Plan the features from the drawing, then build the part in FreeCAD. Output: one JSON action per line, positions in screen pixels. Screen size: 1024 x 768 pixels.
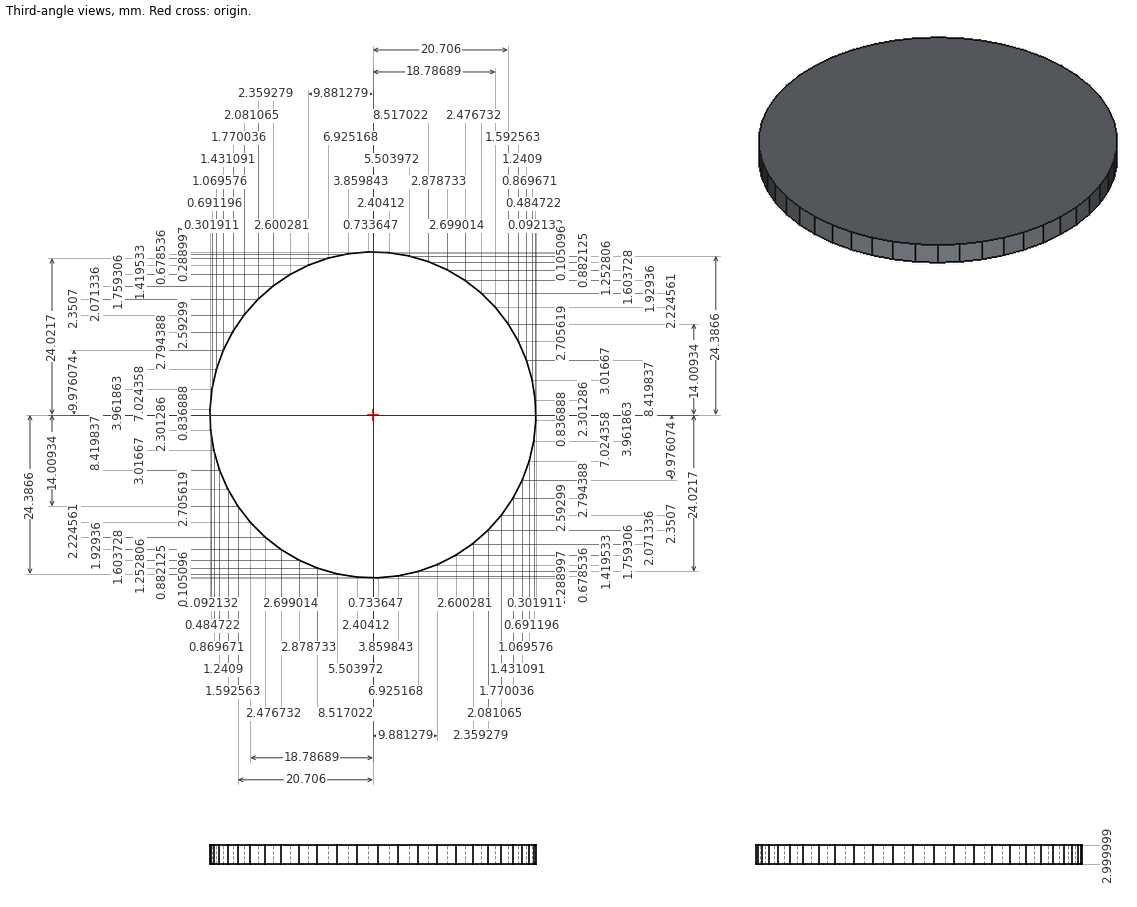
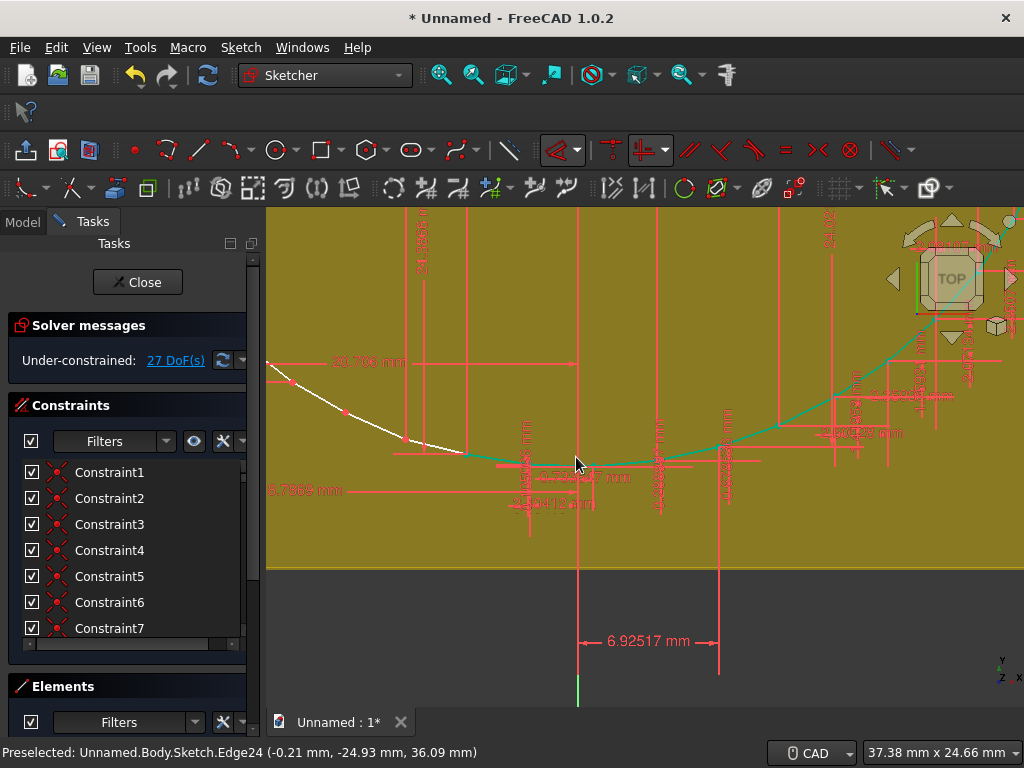
{"action": "scroll", "coordinate": [576, 671], "scroll_direction": "down", "scroll_amount": 6}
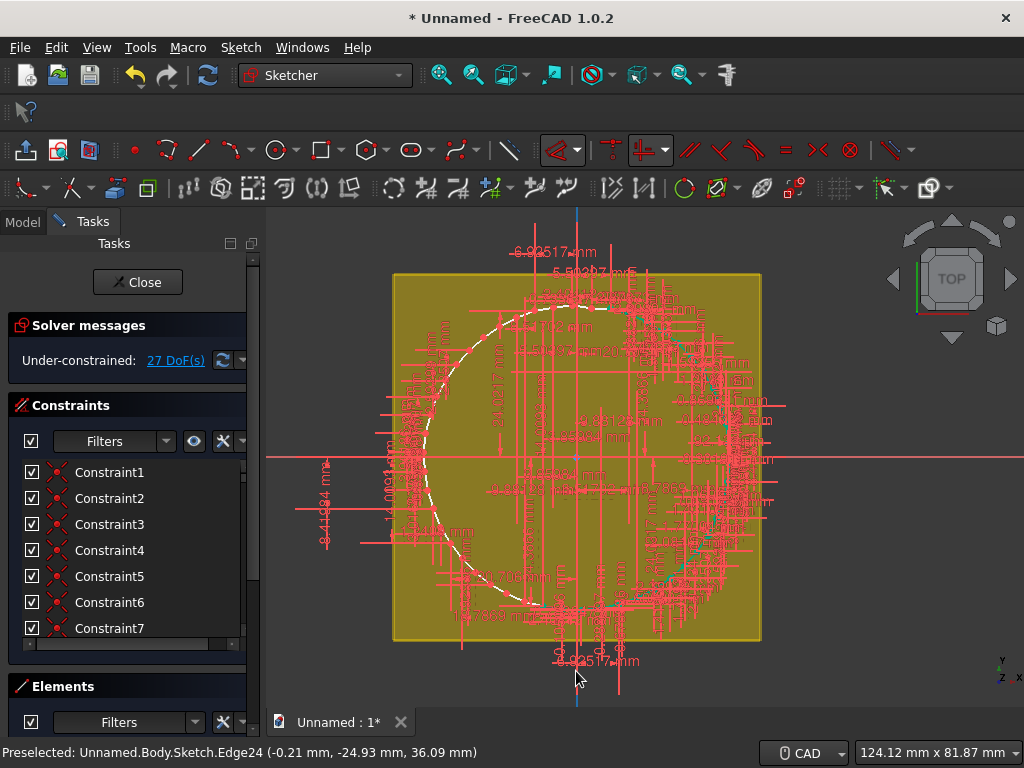
{"action": "scroll", "coordinate": [538, 605], "scroll_direction": "up", "scroll_amount": 10}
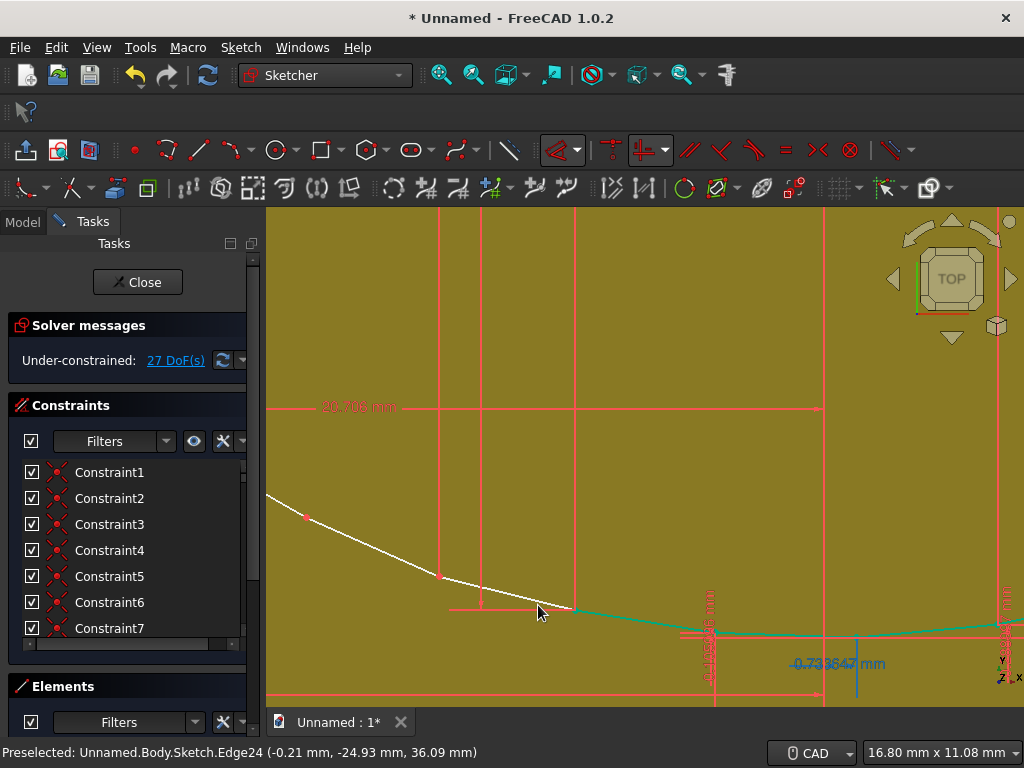
{"action": "left_click", "coordinate": [534, 600]}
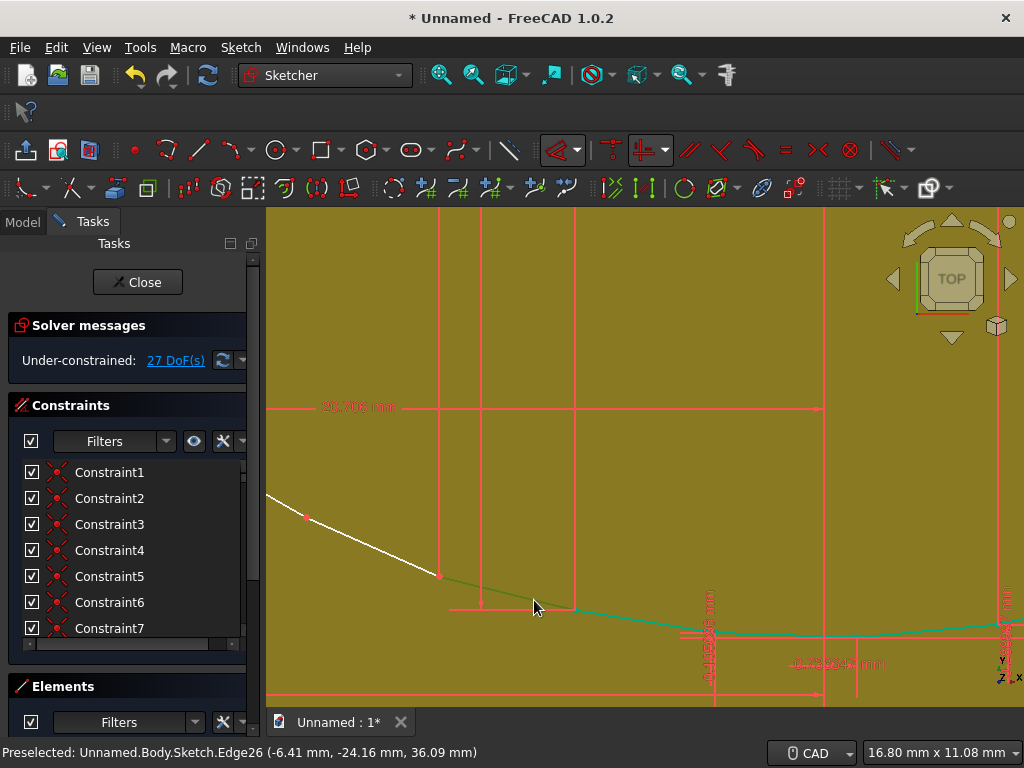
{"action": "left_click", "coordinate": [580, 150]}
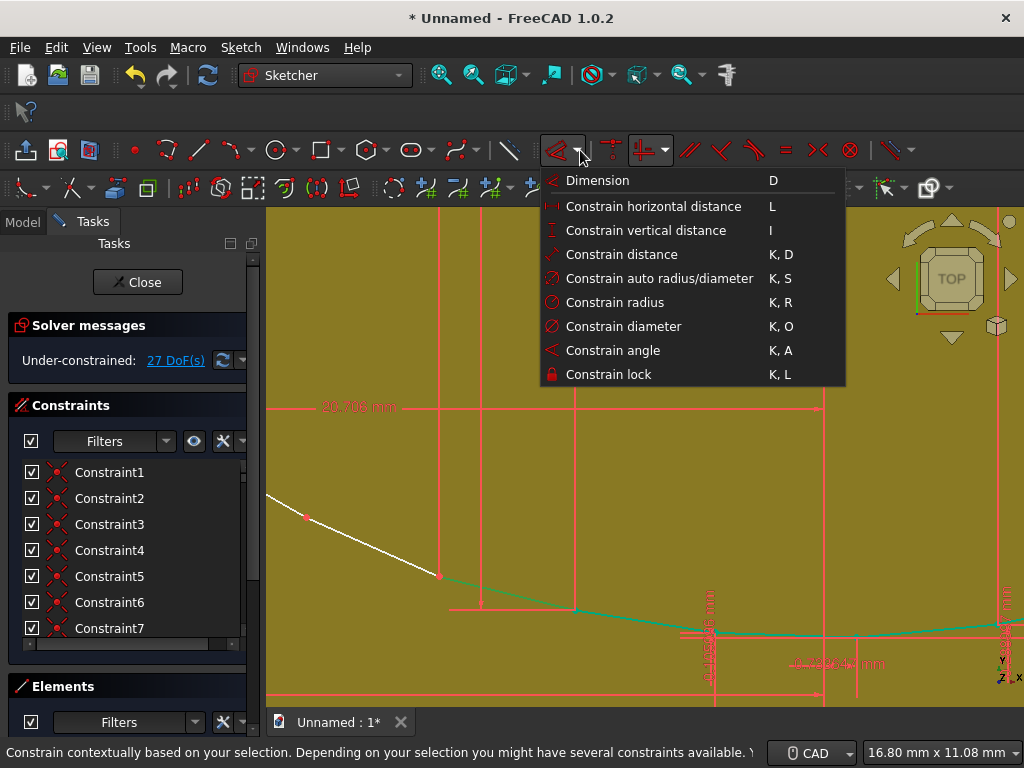
{"action": "left_click", "coordinate": [693, 230]}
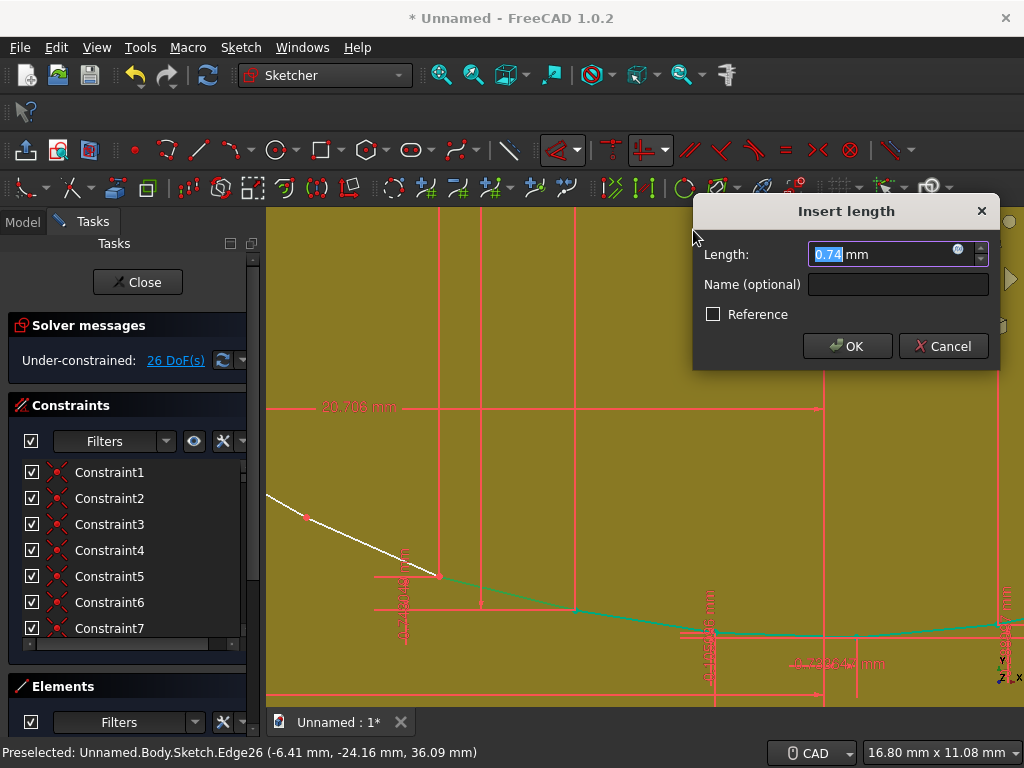
{"action": "type", "text": "0.882125"}
{"action": "key", "text": "Return"}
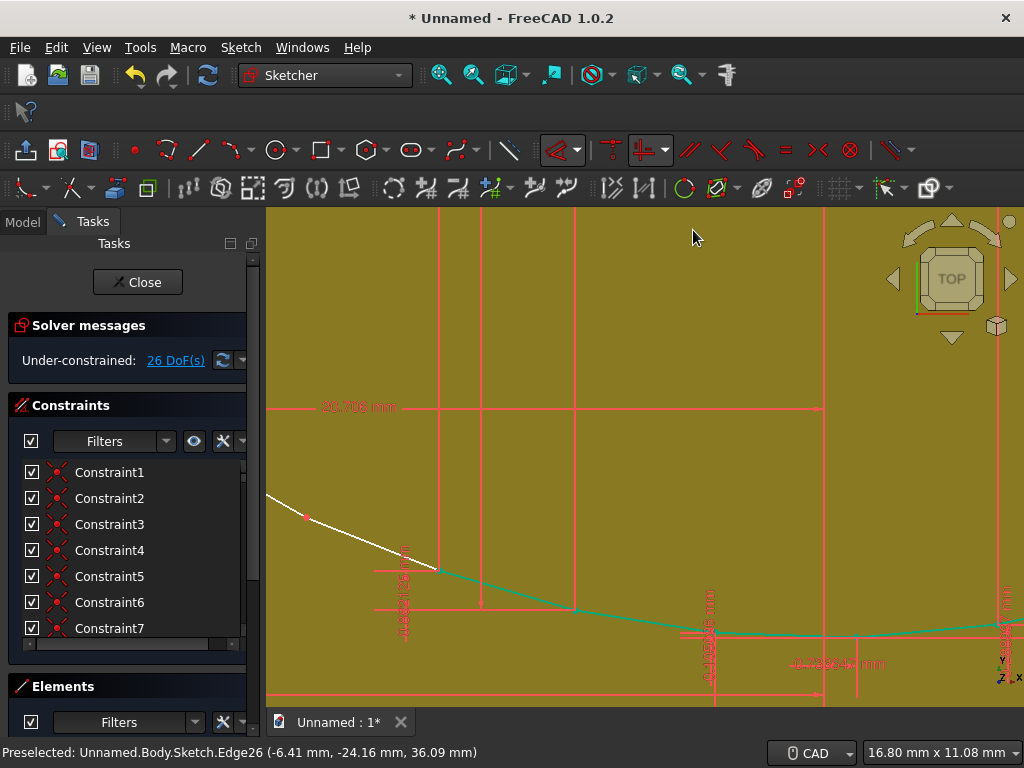
{"action": "scroll", "coordinate": [538, 605], "scroll_direction": "down", "scroll_amount": 10}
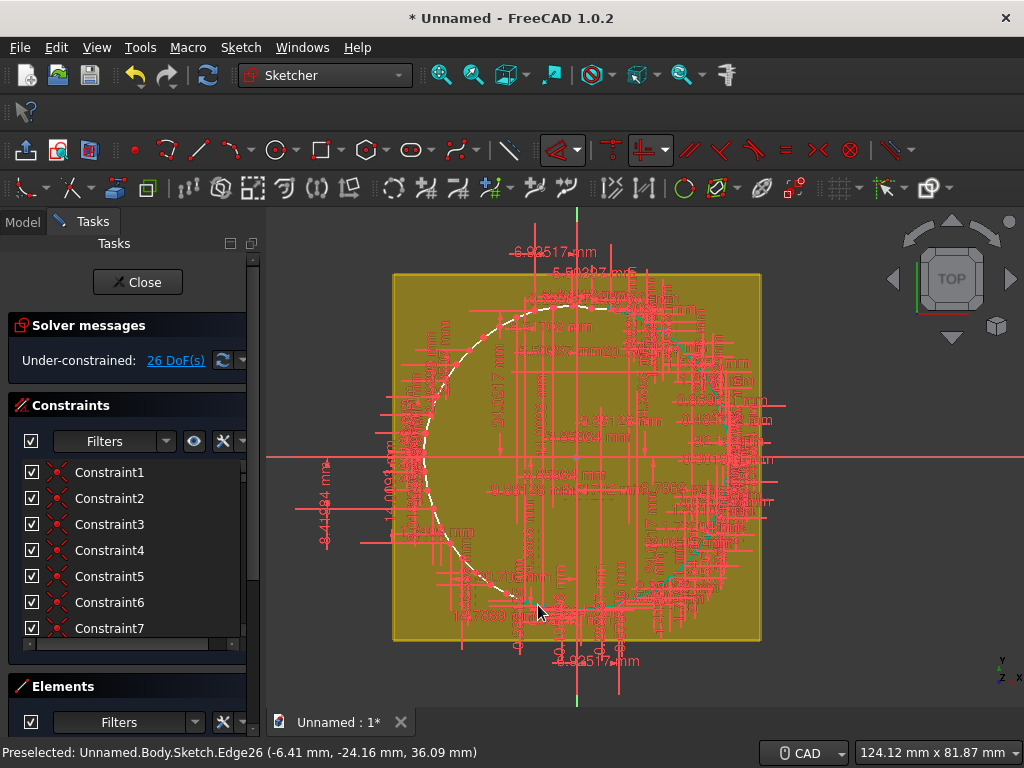
{"action": "scroll", "coordinate": [520, 599], "scroll_direction": "up", "scroll_amount": 5}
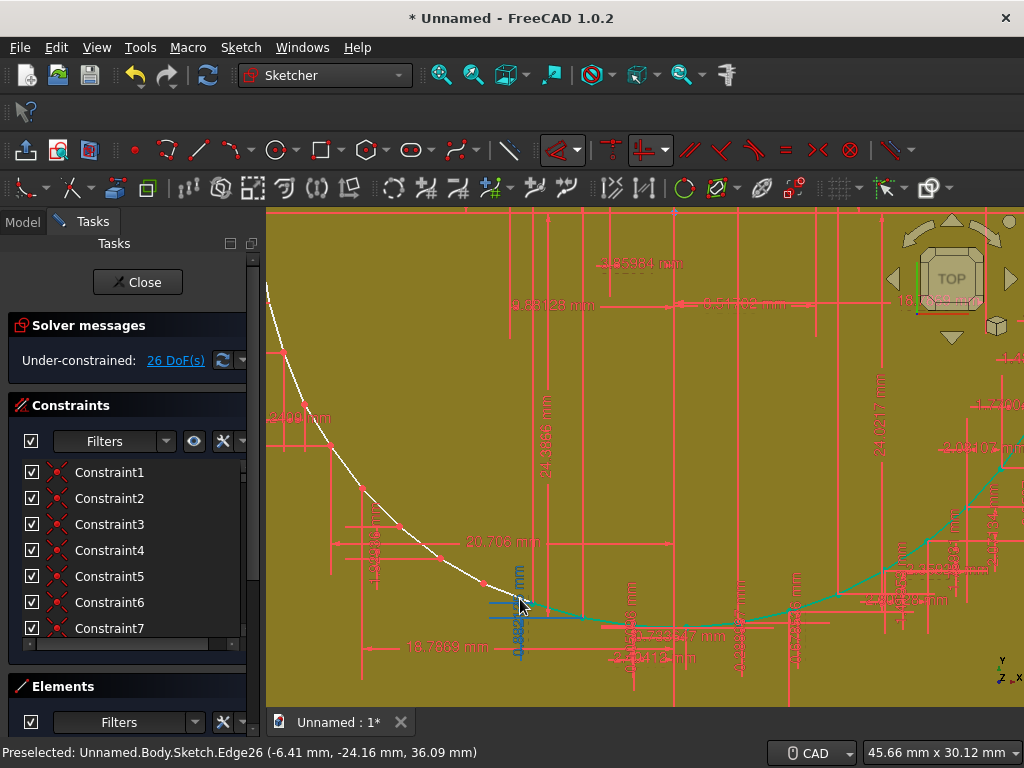
{"action": "left_click", "coordinate": [499, 590]}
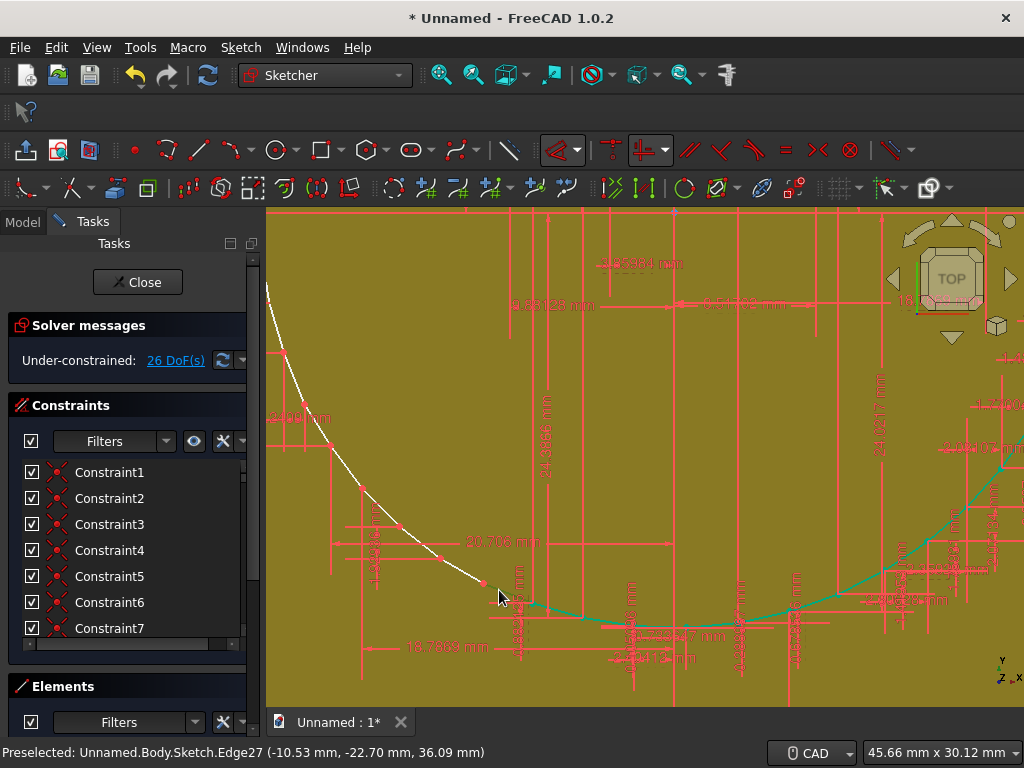
{"action": "left_click", "coordinate": [580, 150]}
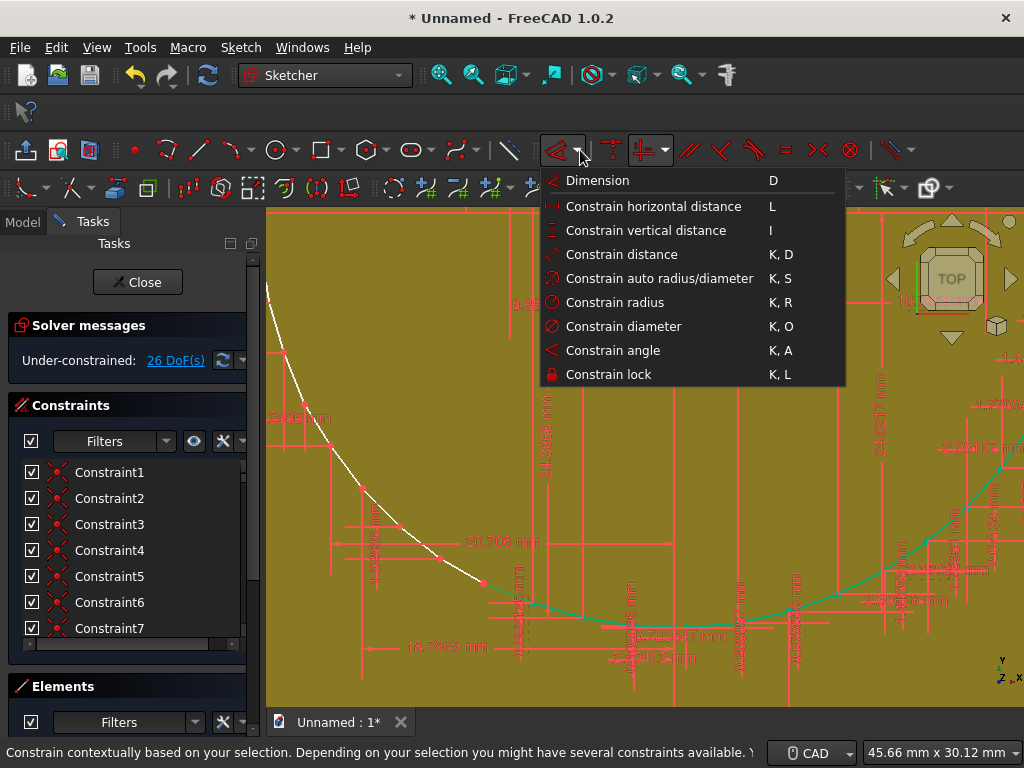
{"action": "left_click", "coordinate": [693, 206]}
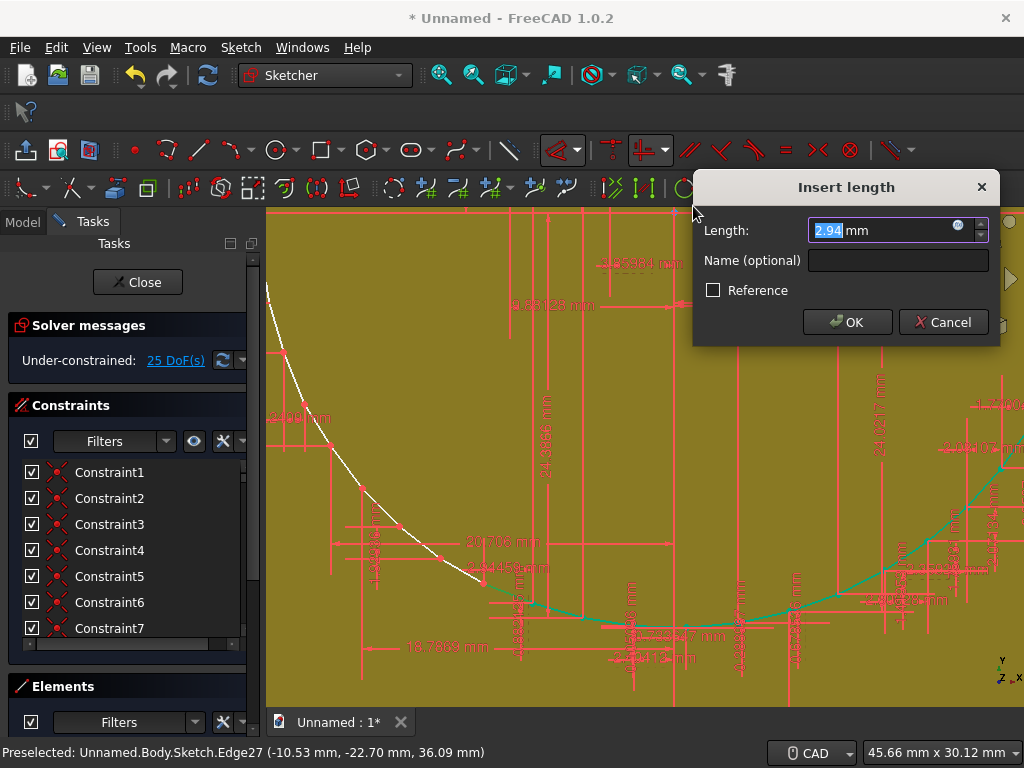
{"action": "type", "text": "2.878733"}
{"action": "key", "text": "Return"}